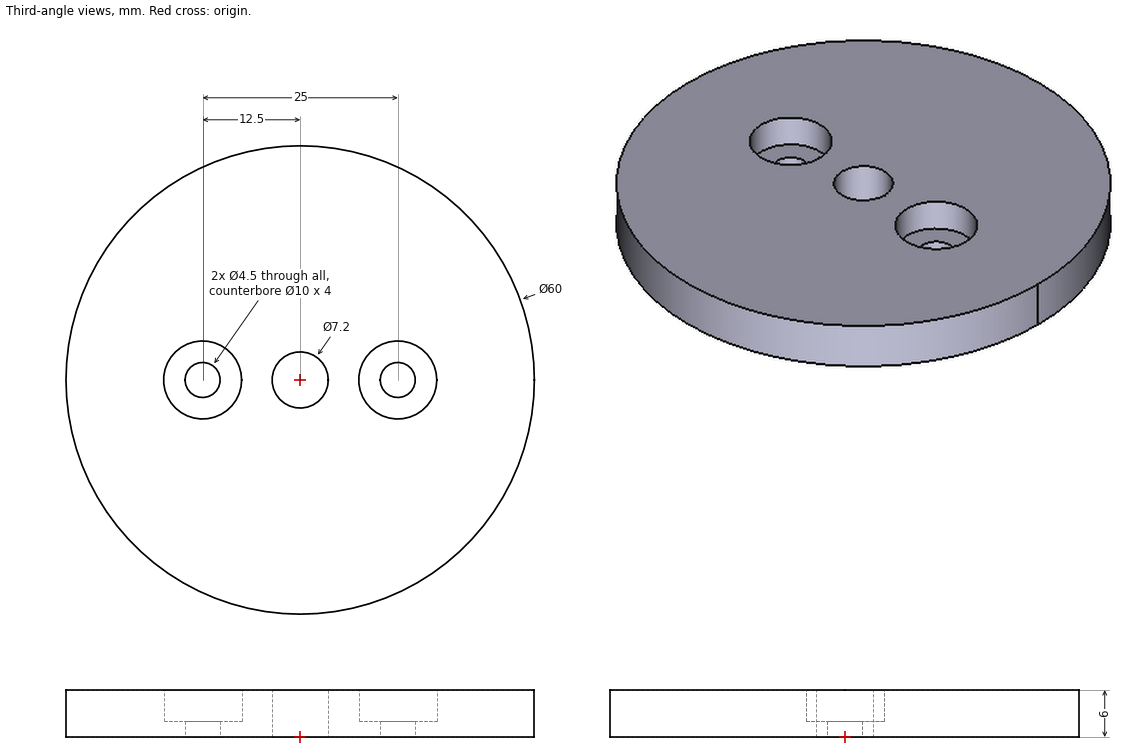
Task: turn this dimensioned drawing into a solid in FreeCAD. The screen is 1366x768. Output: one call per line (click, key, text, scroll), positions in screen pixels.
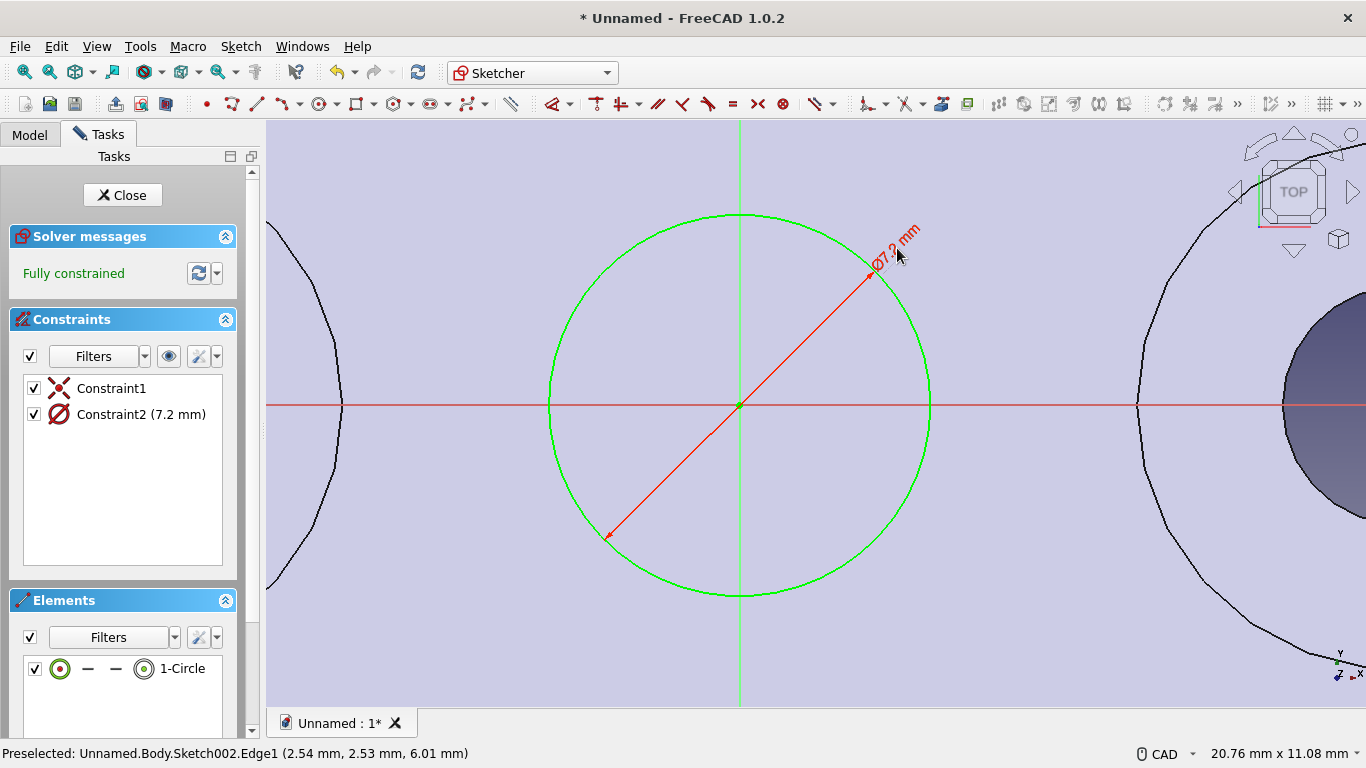
click(123, 195)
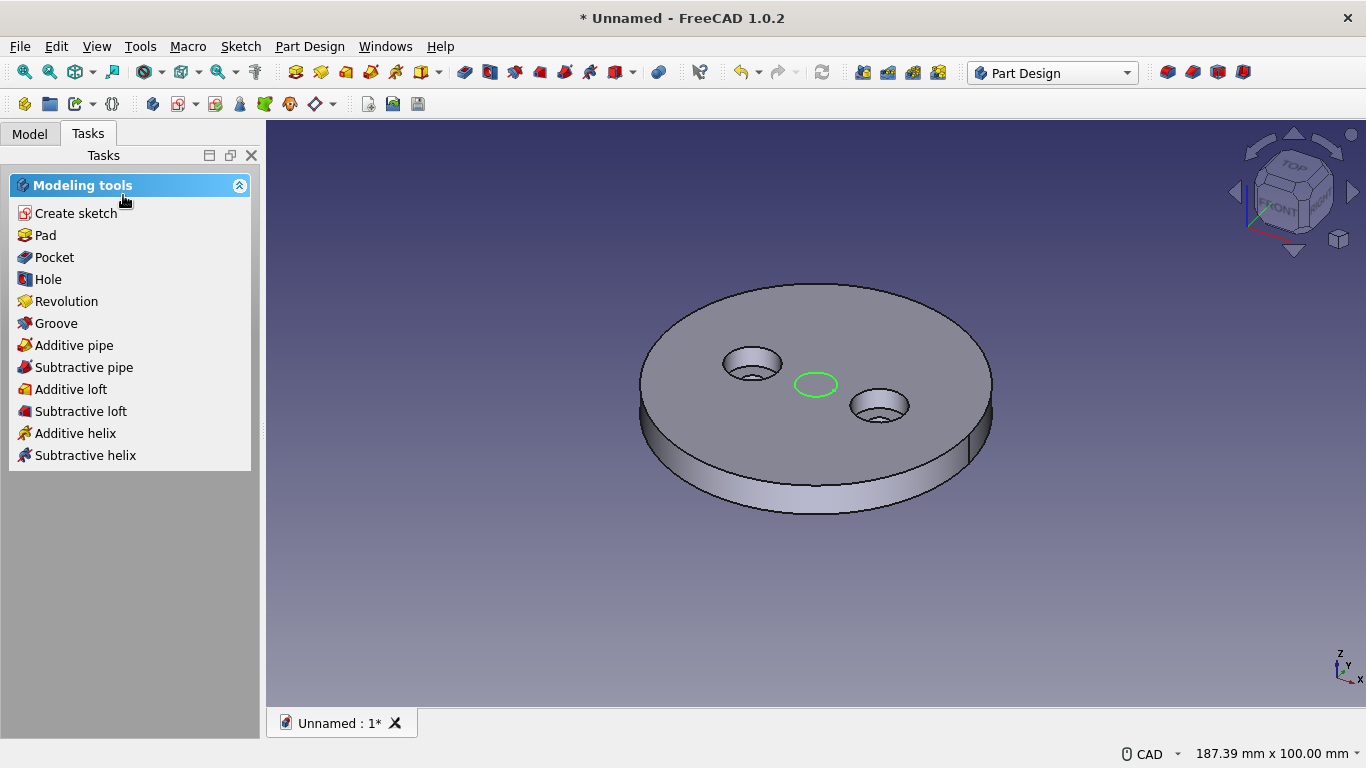
click(465, 72)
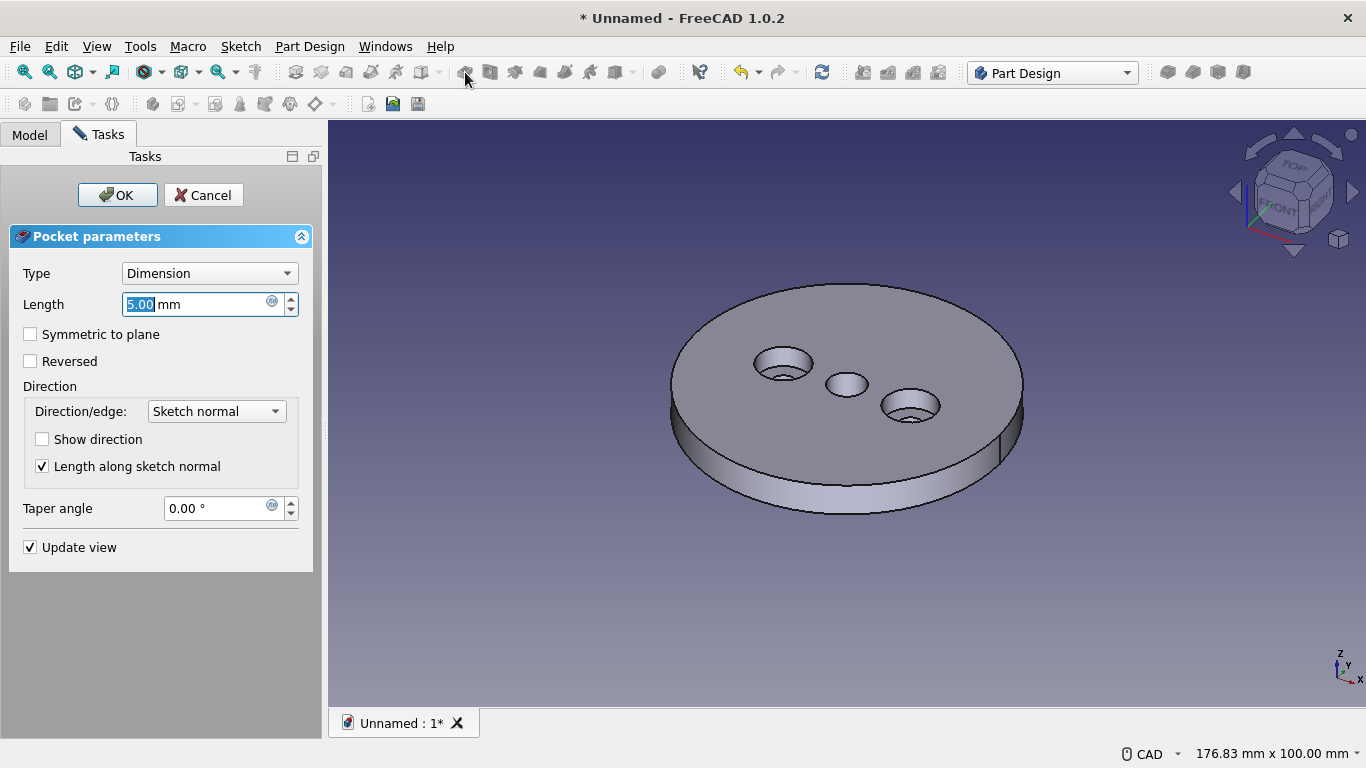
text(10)
key(Tab)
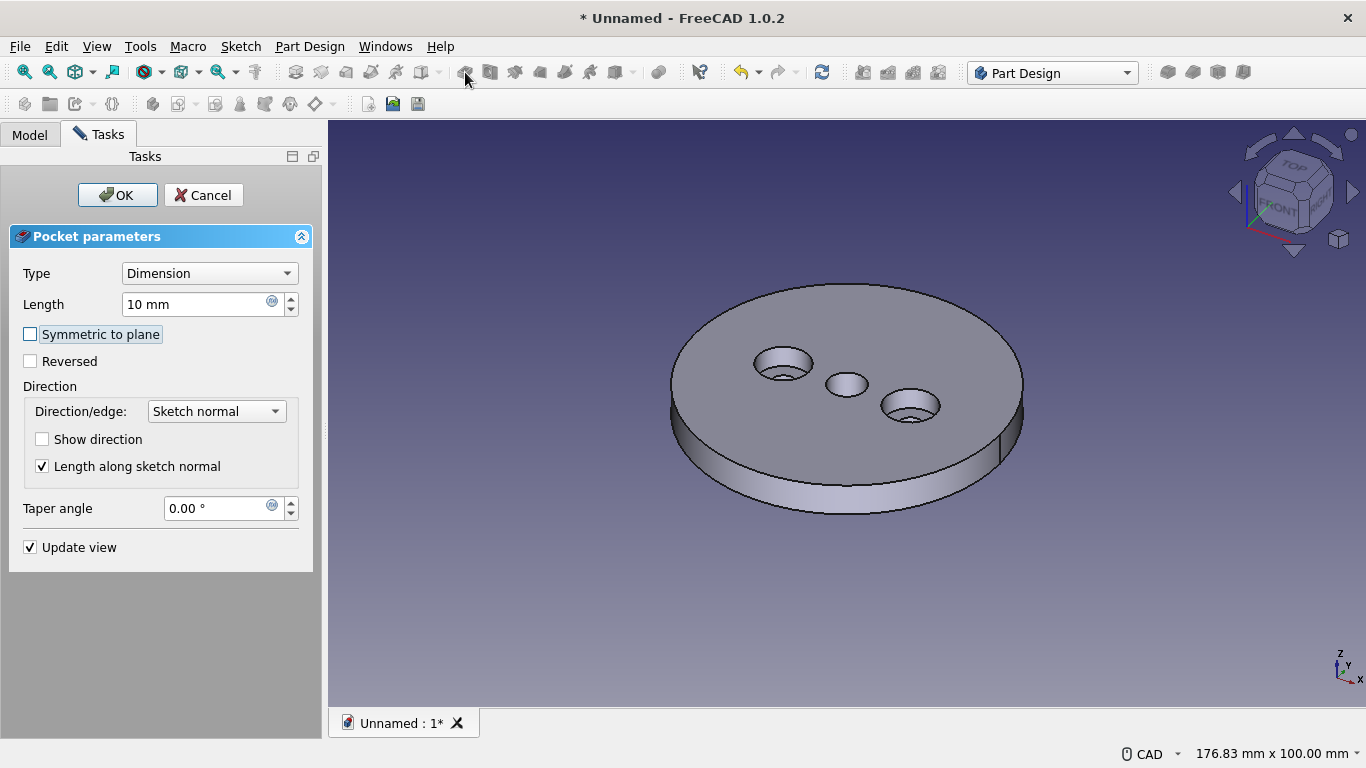
click(118, 195)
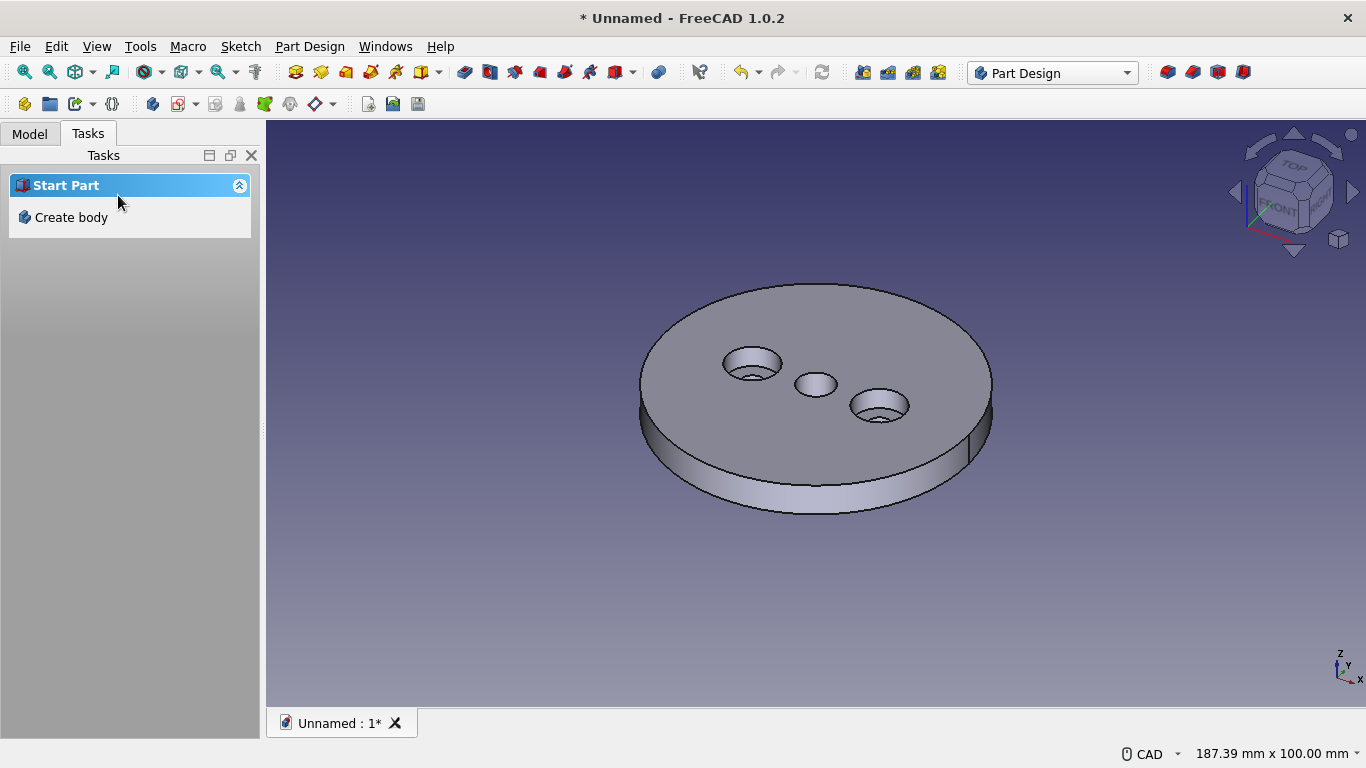
key(0)